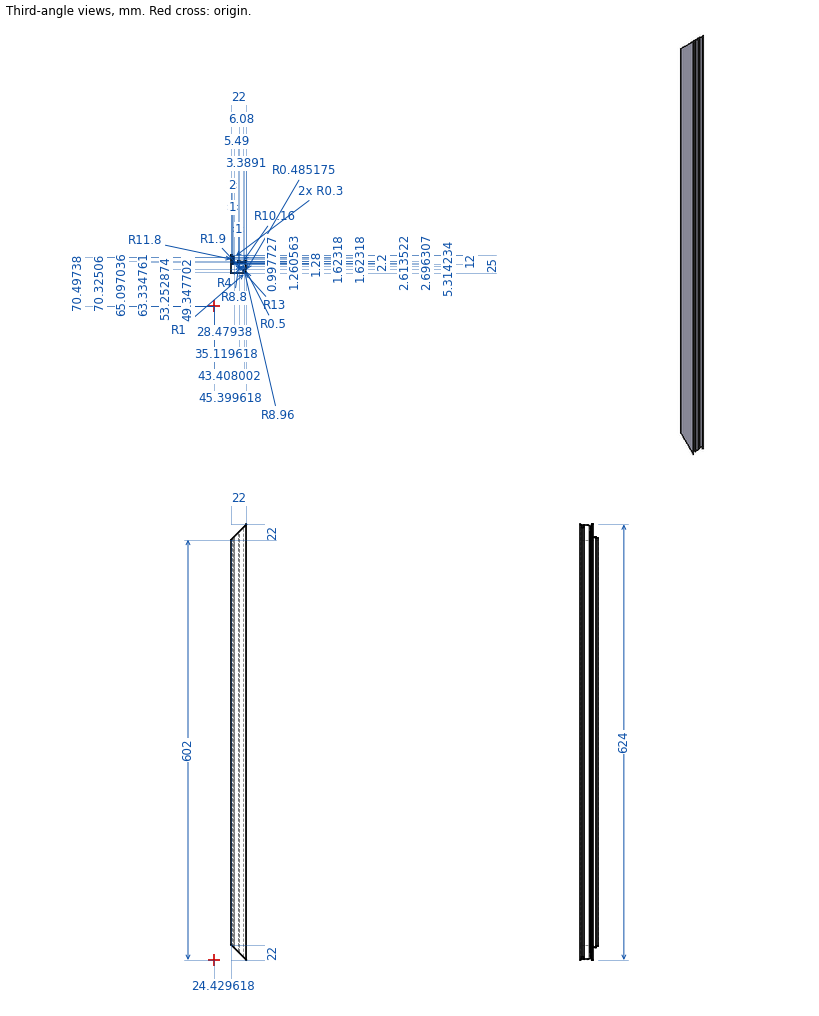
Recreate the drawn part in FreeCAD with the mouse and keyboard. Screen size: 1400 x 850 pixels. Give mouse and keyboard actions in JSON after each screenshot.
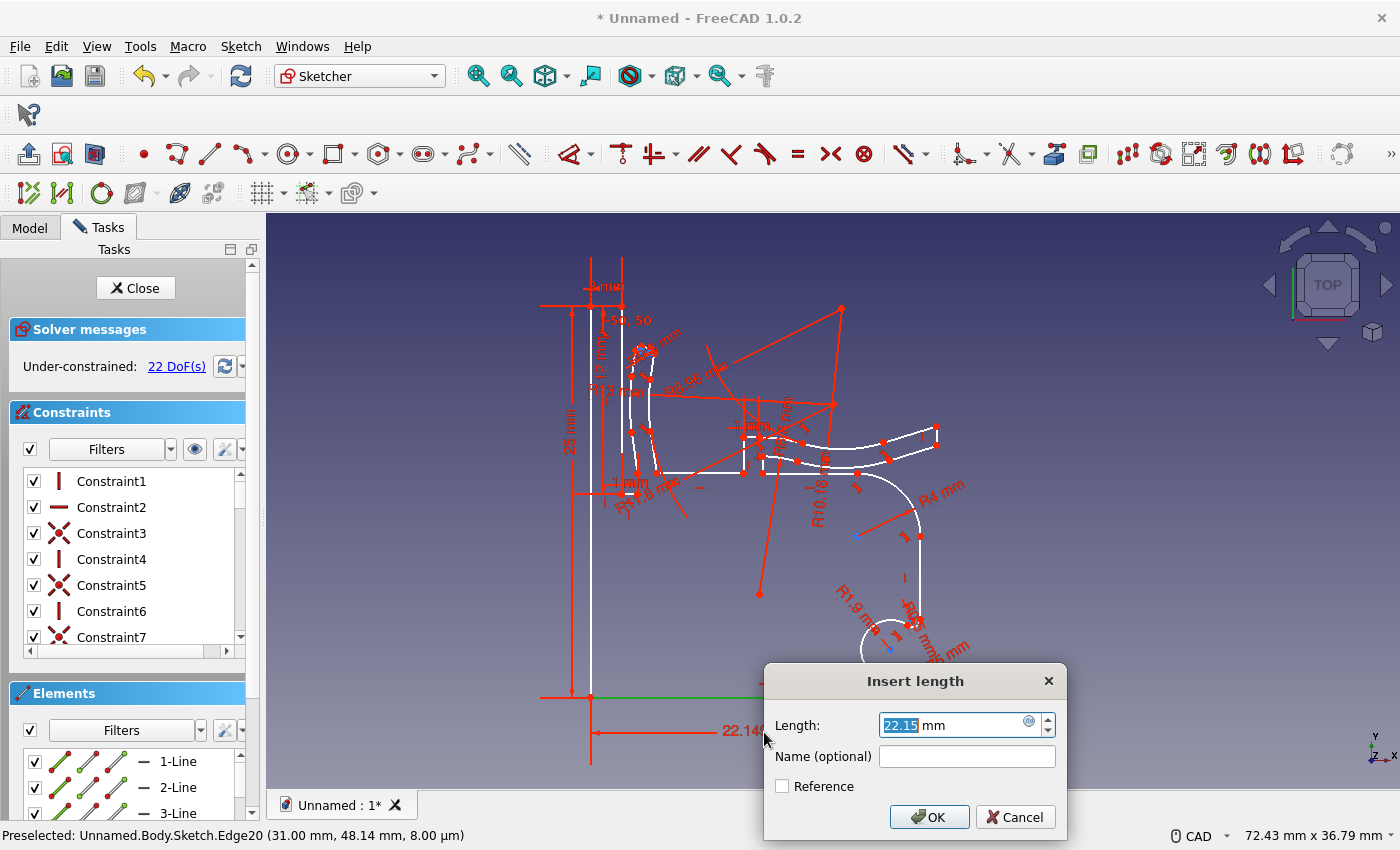
{"action": "type", "text": "22"}
{"action": "key", "text": "Return"}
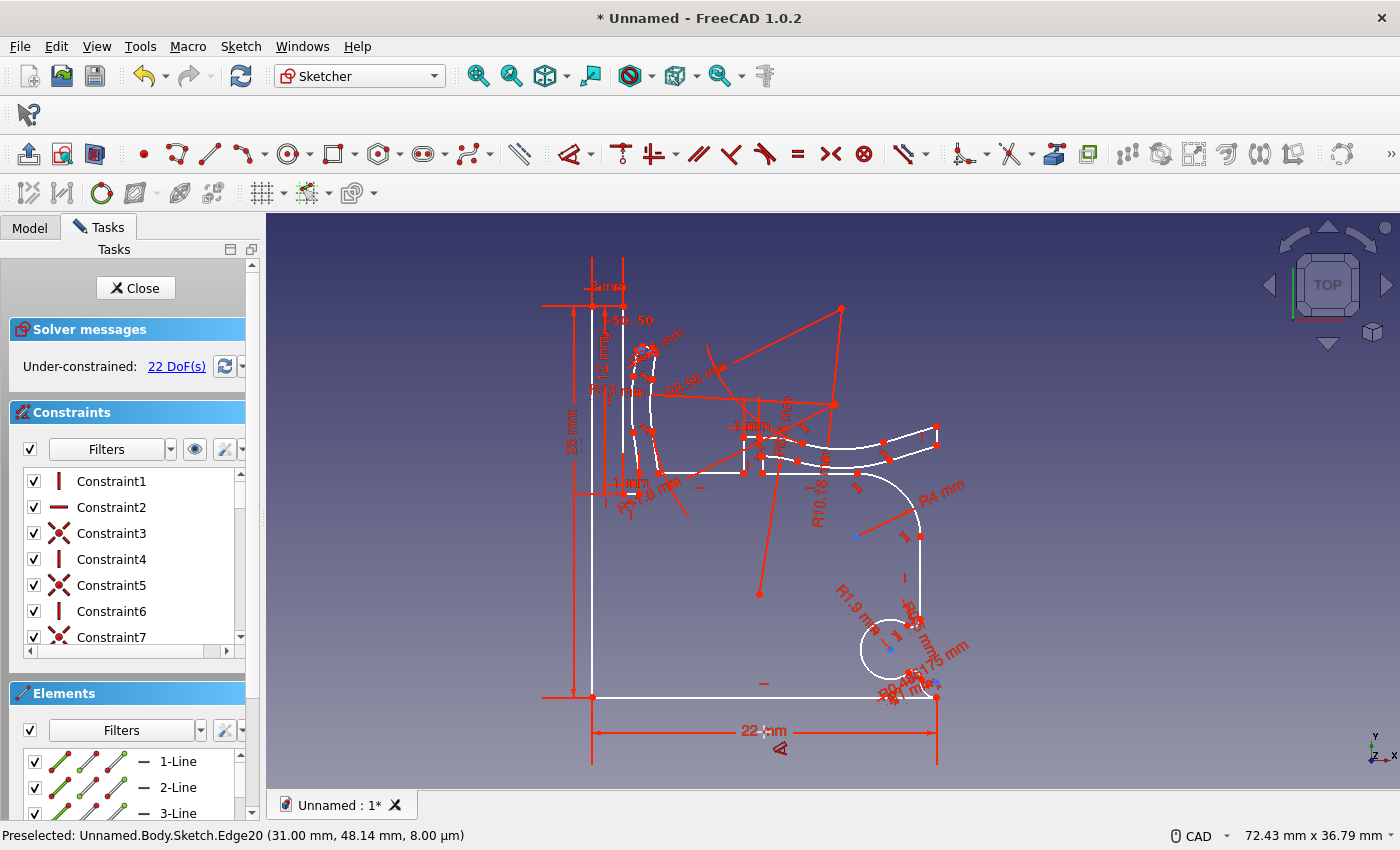
{"action": "scroll", "coordinate": [744, 448], "scroll_direction": "up", "scroll_amount": 2}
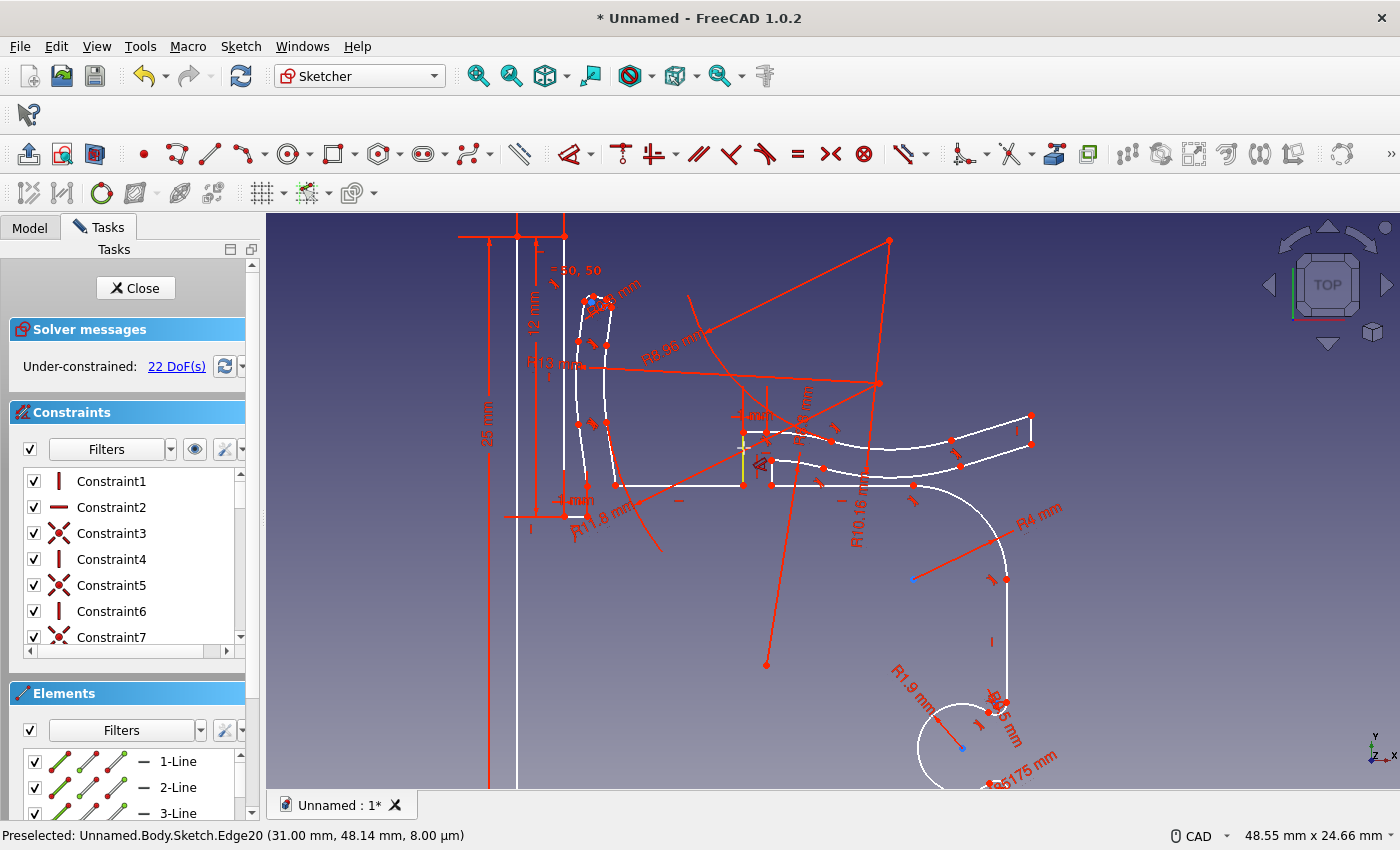
{"action": "left_click", "coordinate": [743, 448]}
{"action": "left_click", "coordinate": [709, 459]}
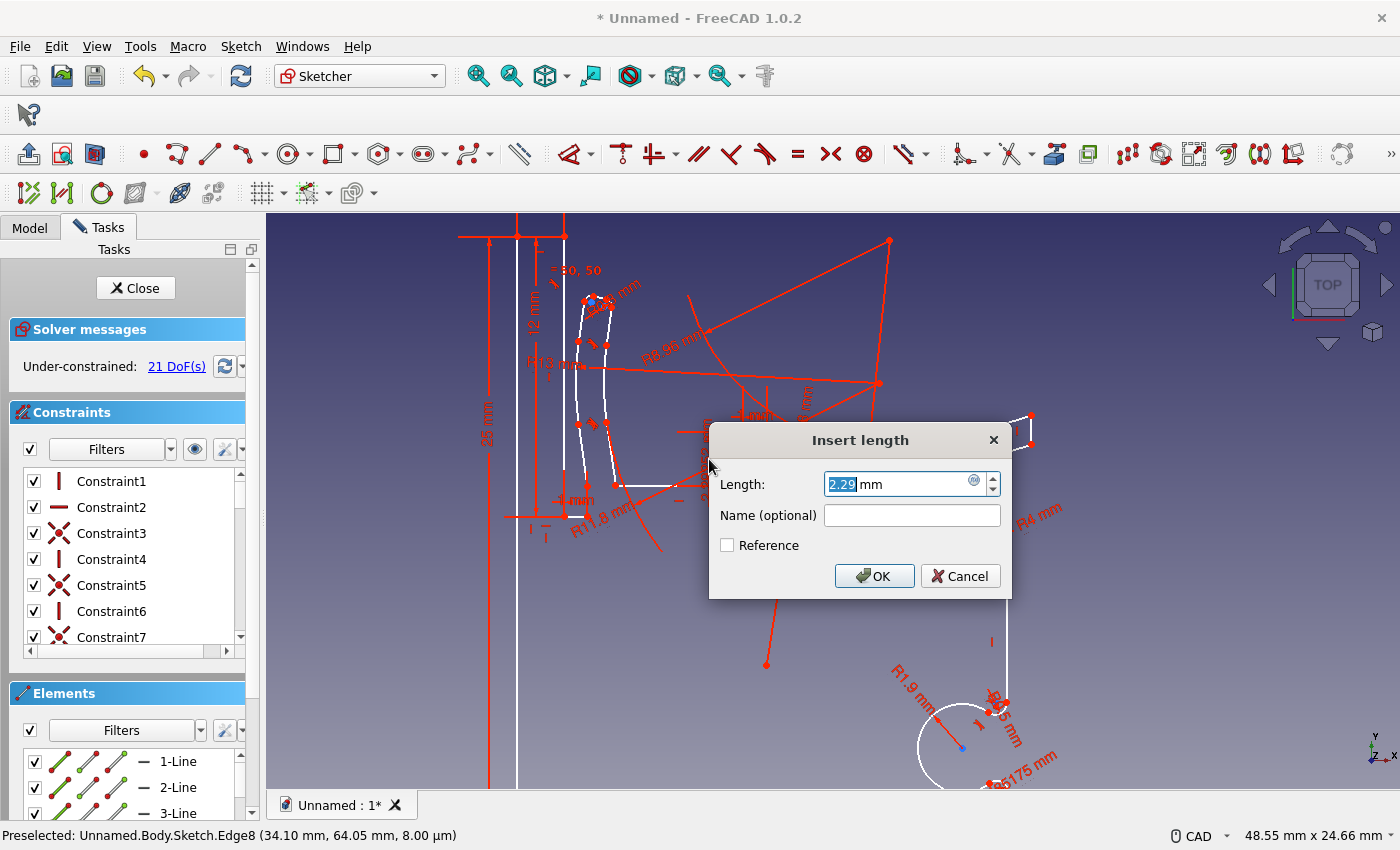
{"action": "type", "text": "2.2"}
{"action": "key", "text": "Return"}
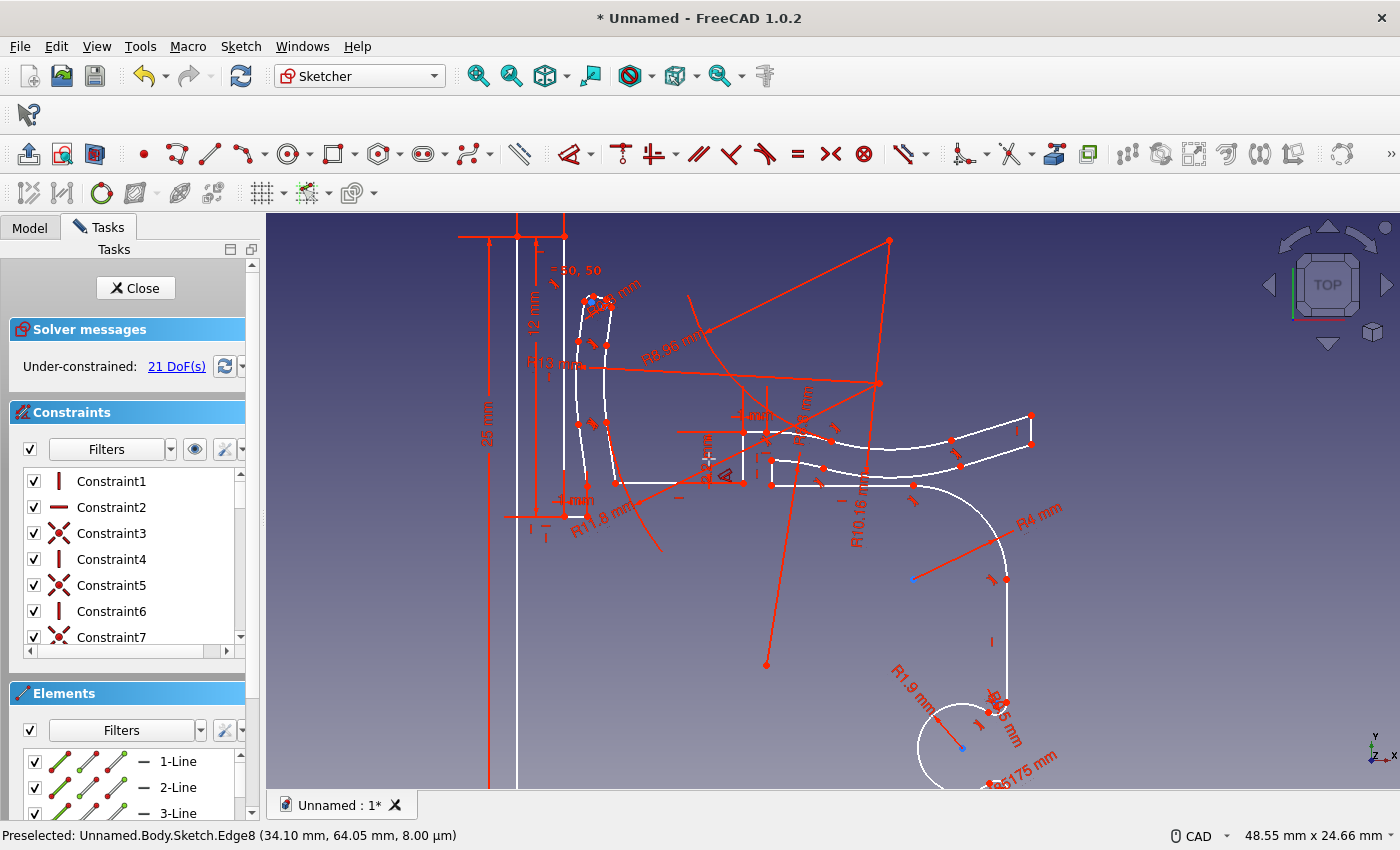
{"action": "scroll", "coordinate": [871, 486], "scroll_direction": "up", "scroll_amount": 3}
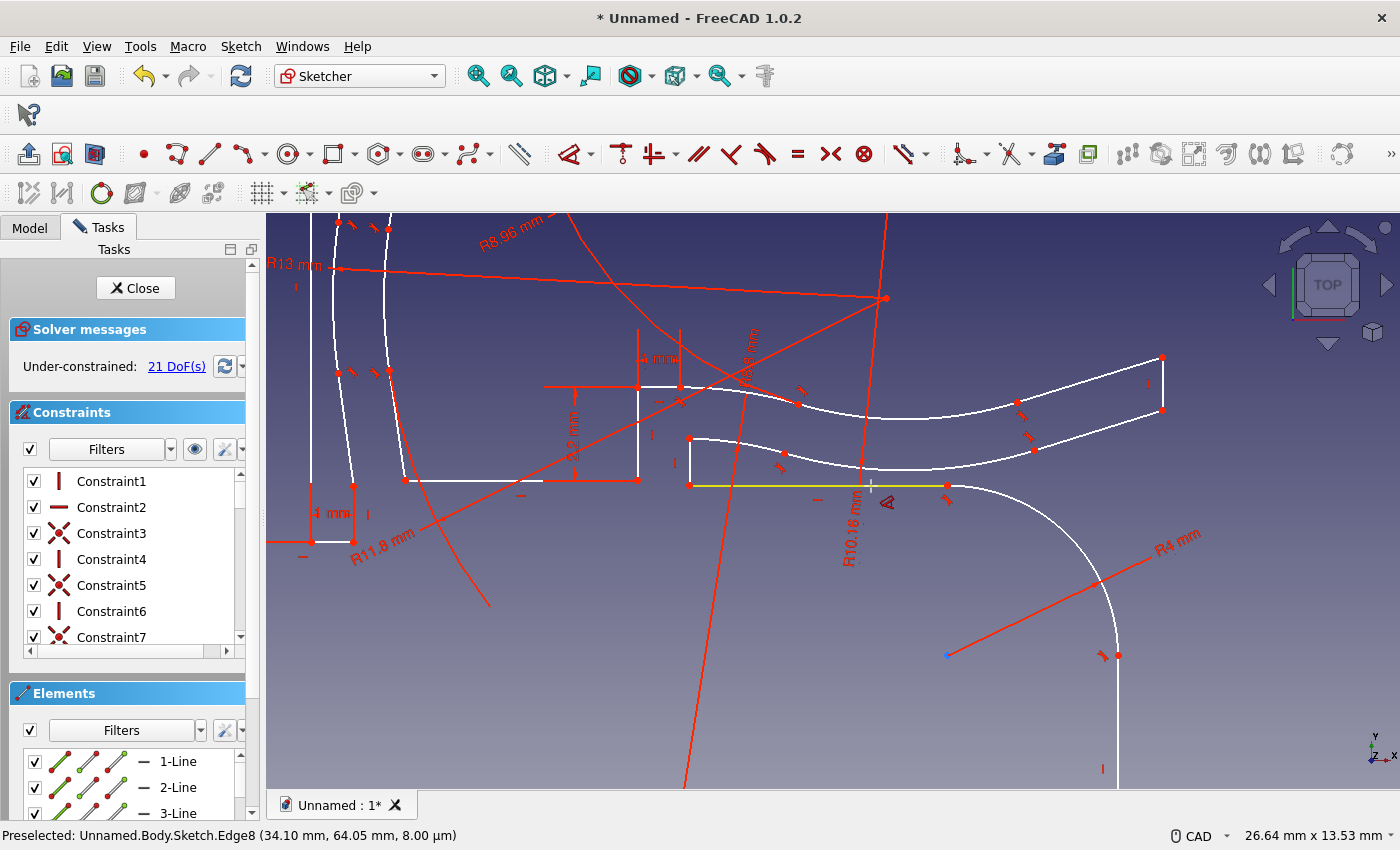
{"action": "left_click", "coordinate": [870, 486]}
{"action": "left_click", "coordinate": [878, 452]}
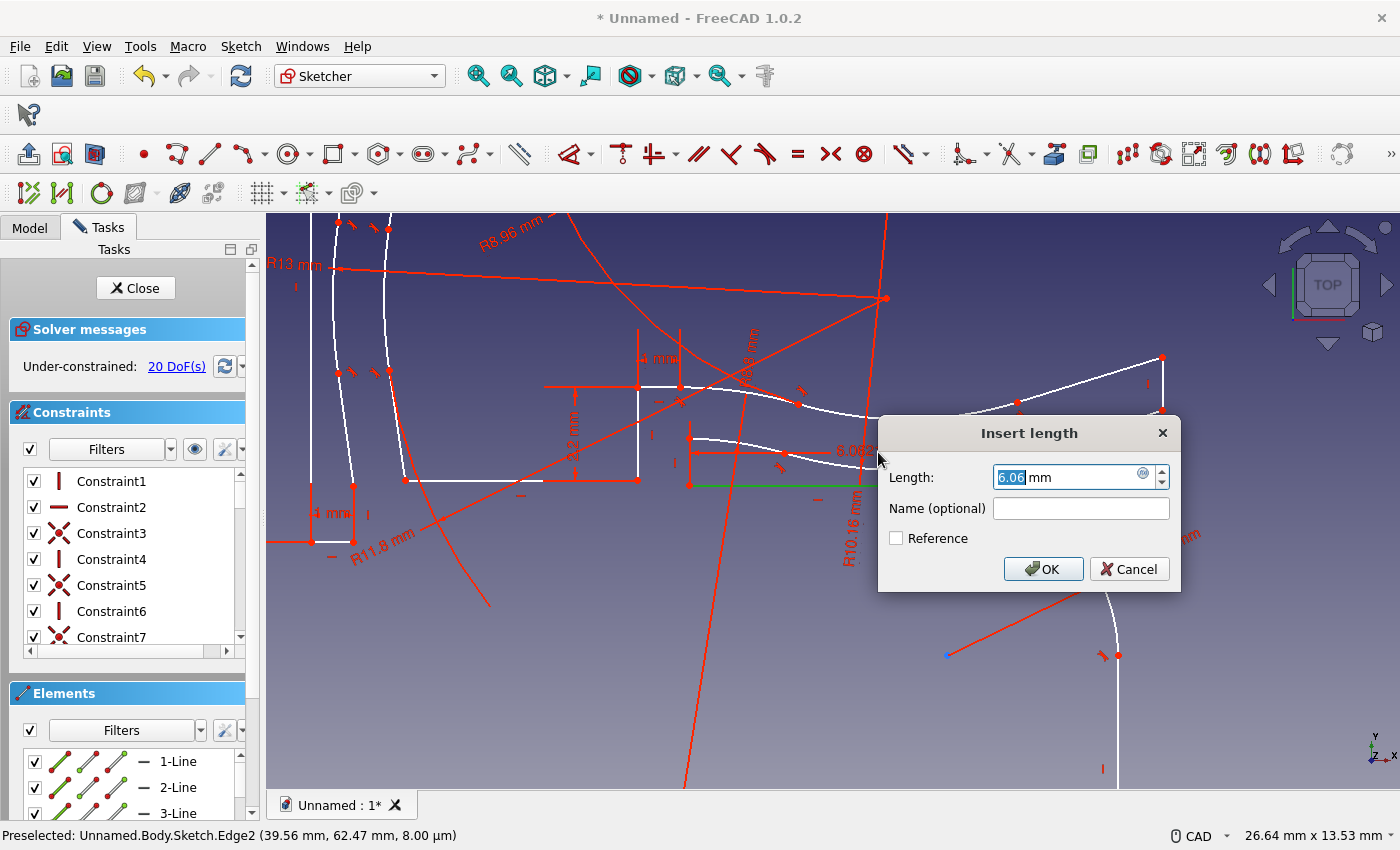
{"action": "type", "text": "6.08"}
{"action": "key", "text": "Return"}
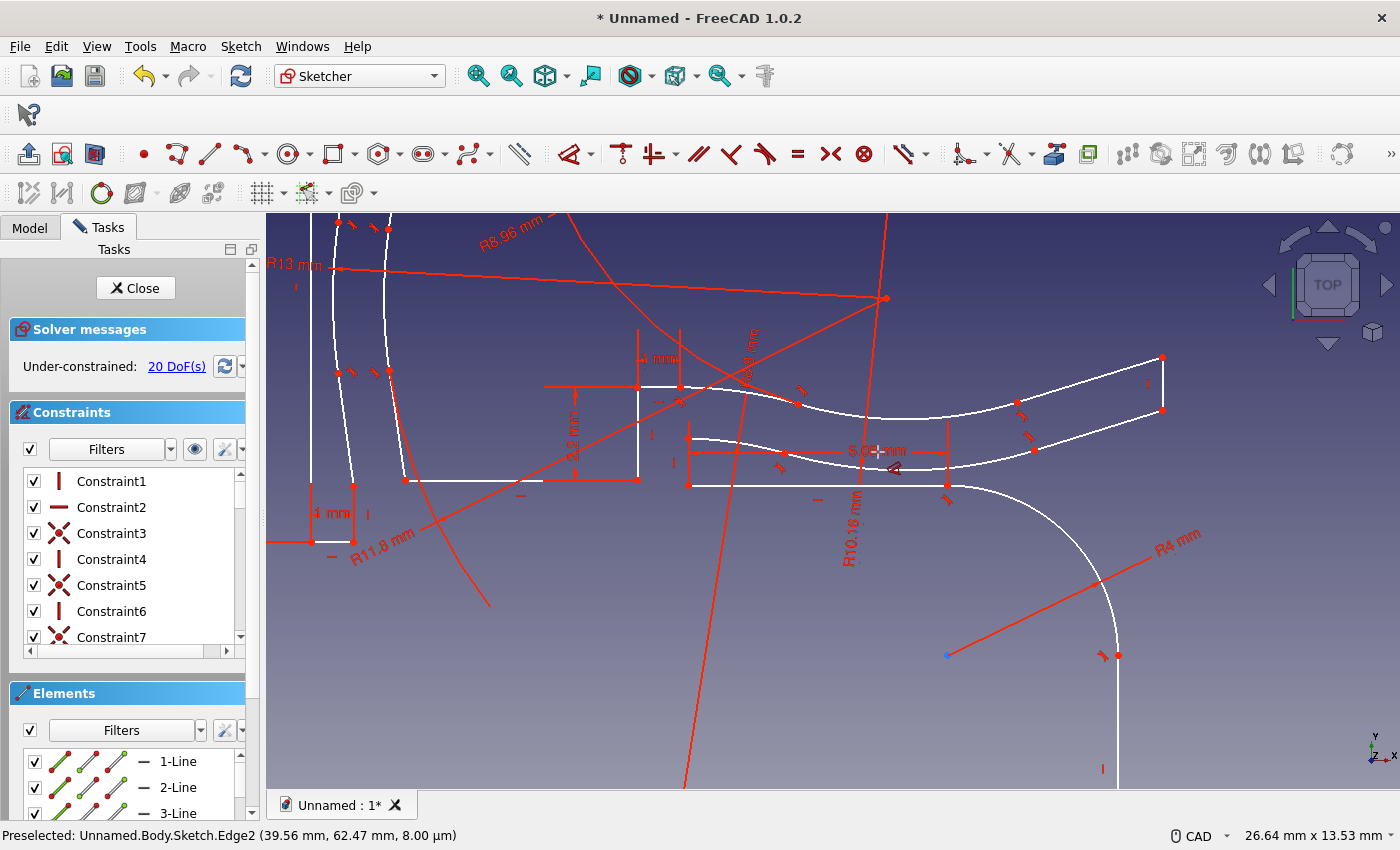
{"action": "left_click", "coordinate": [568, 481]}
{"action": "left_click", "coordinate": [468, 447]}